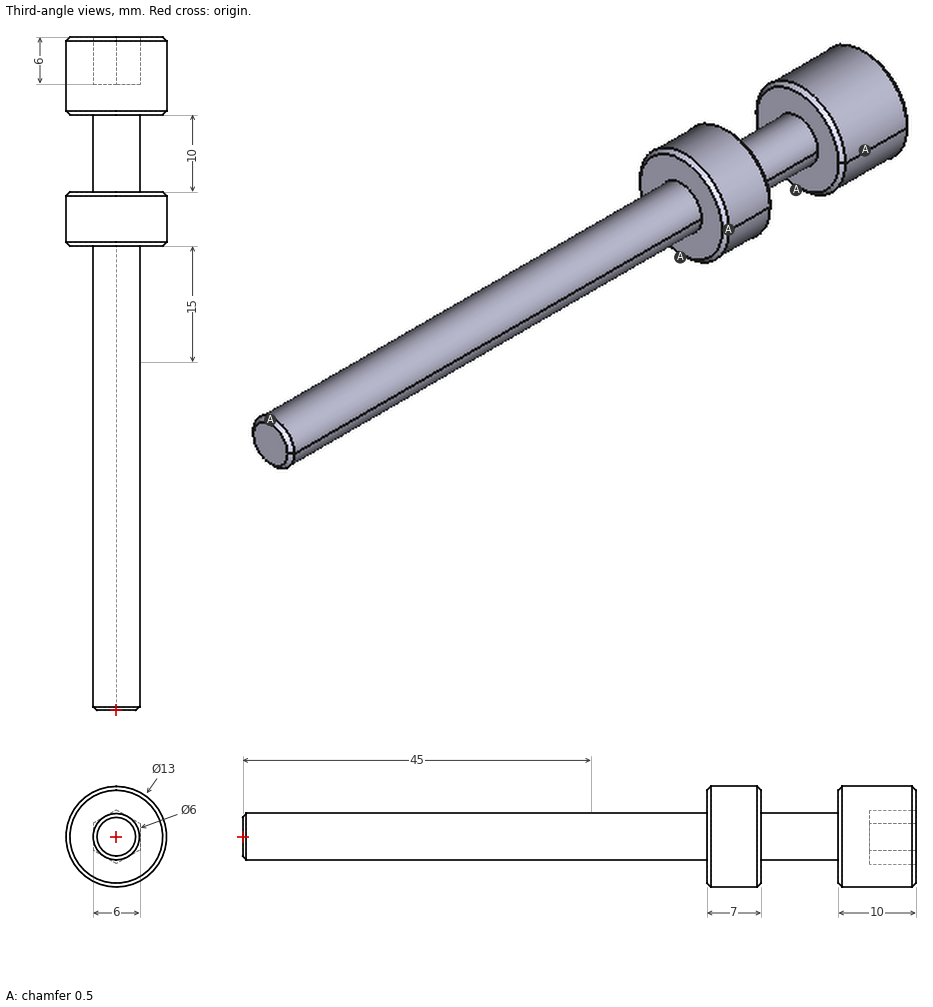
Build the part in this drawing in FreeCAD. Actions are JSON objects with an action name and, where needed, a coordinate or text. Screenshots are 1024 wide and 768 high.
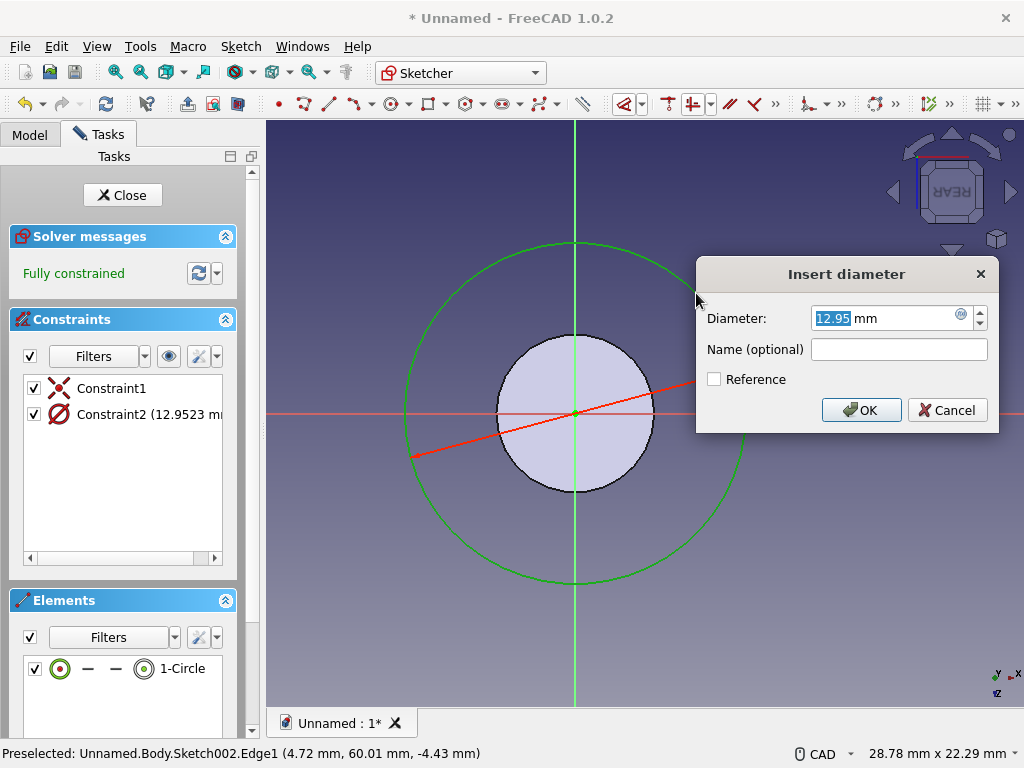
{"action": "type", "text": "13"}
{"action": "key", "text": "Return"}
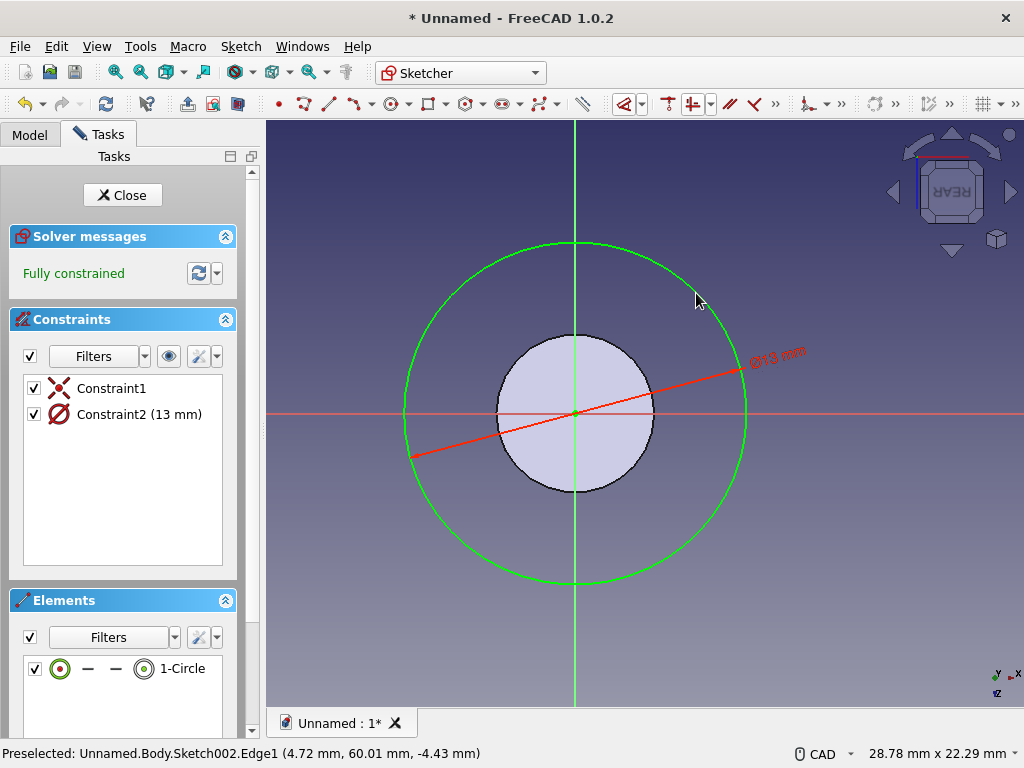
{"action": "left_click", "coordinate": [123, 195]}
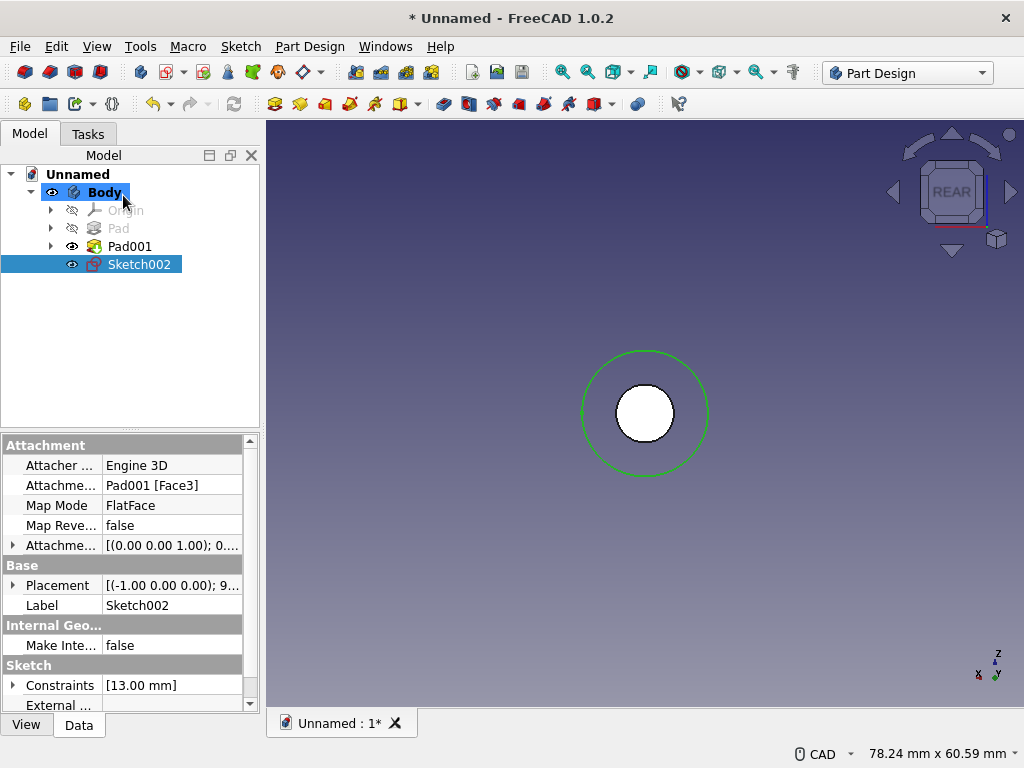
{"action": "left_click", "coordinate": [275, 104]}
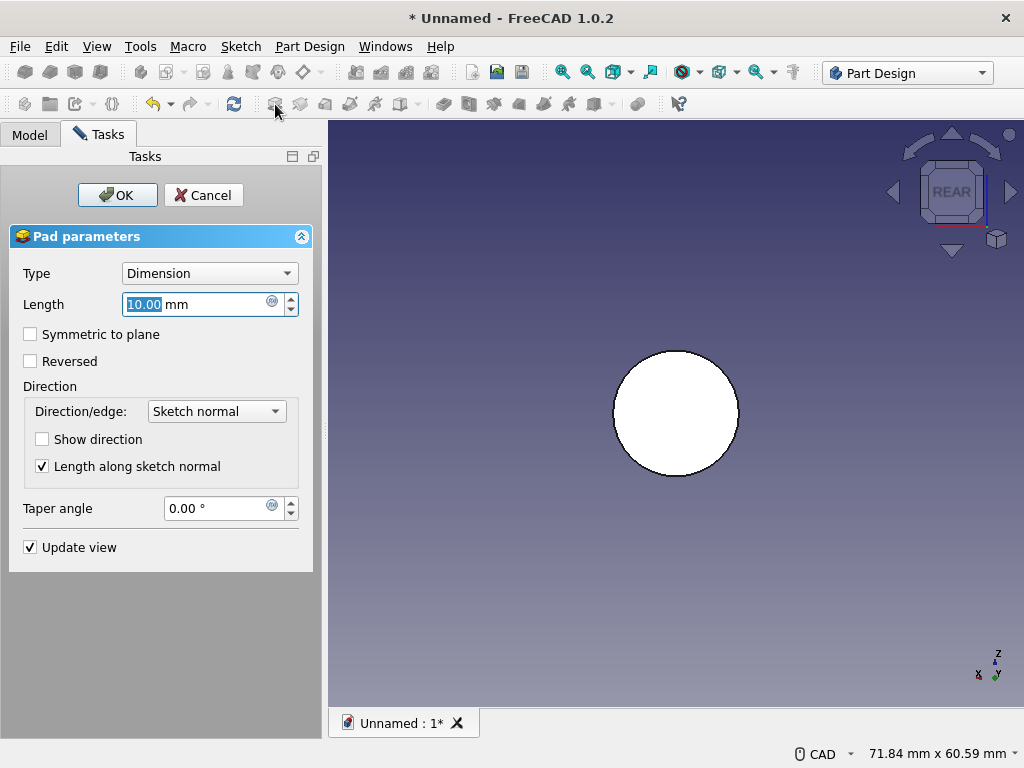
{"action": "type", "text": "7"}
{"action": "key", "text": "Tab"}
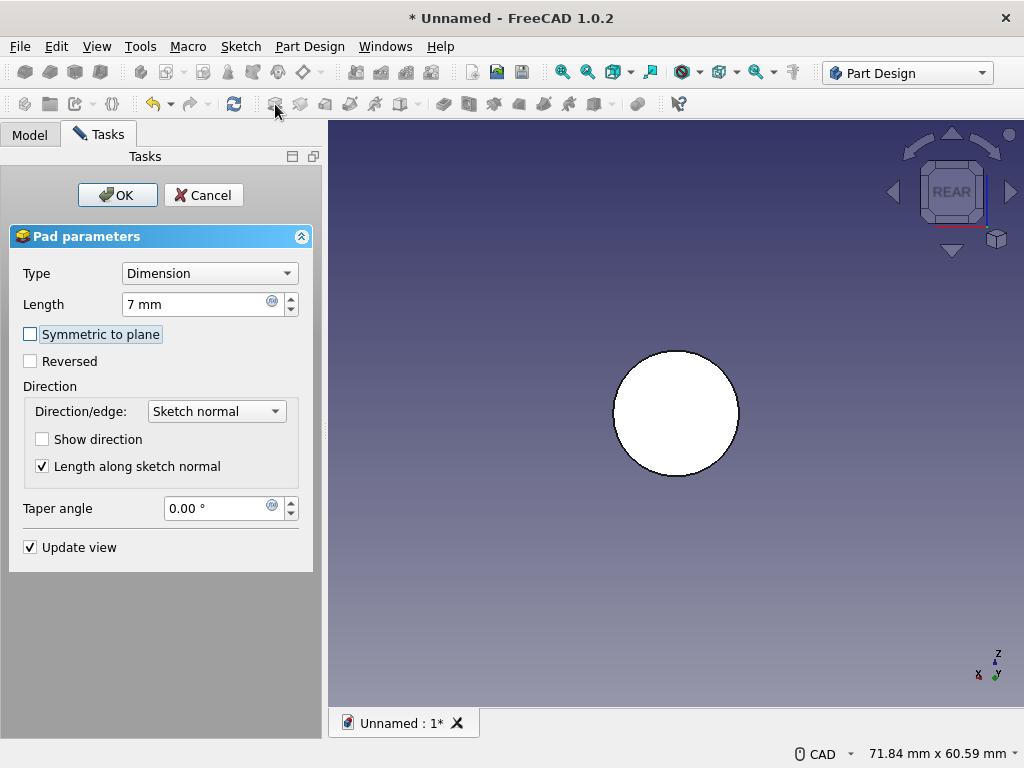
{"action": "left_click", "coordinate": [118, 195]}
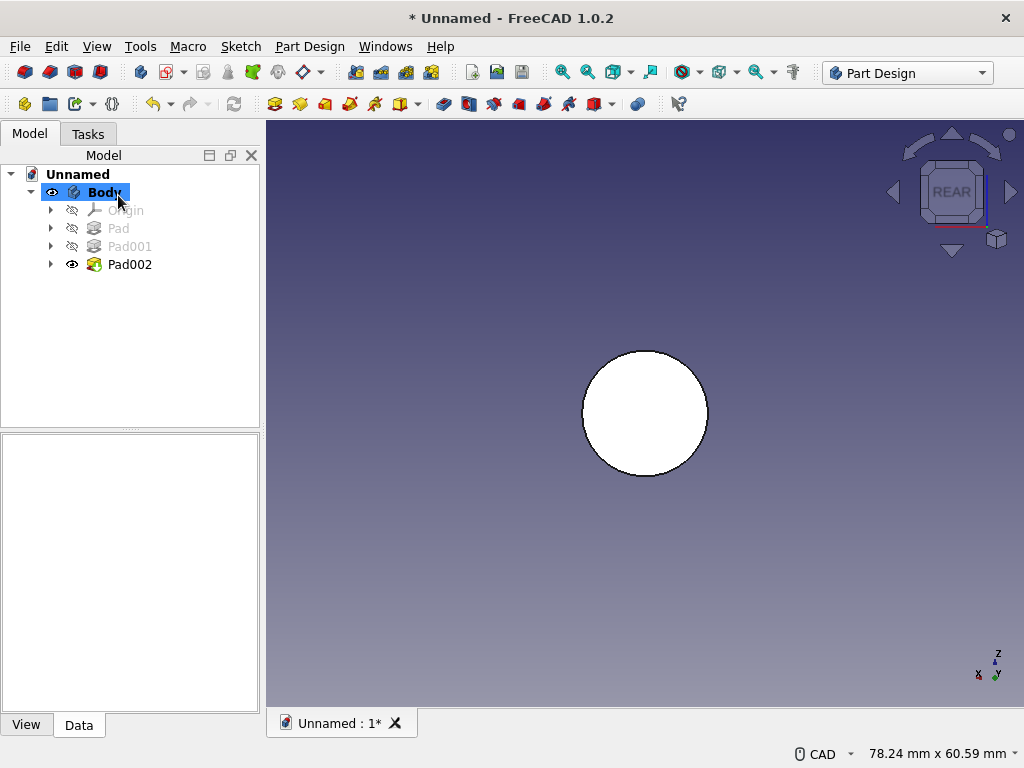
{"action": "key", "text": "v f"}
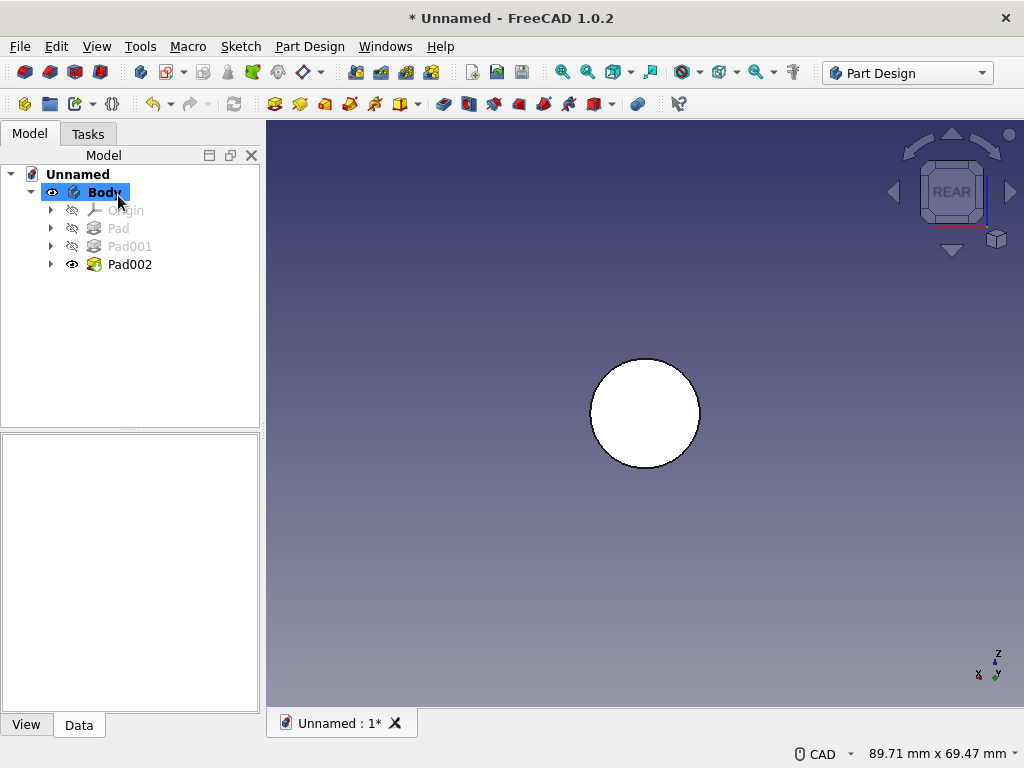
{"action": "left_click", "coordinate": [645, 412]}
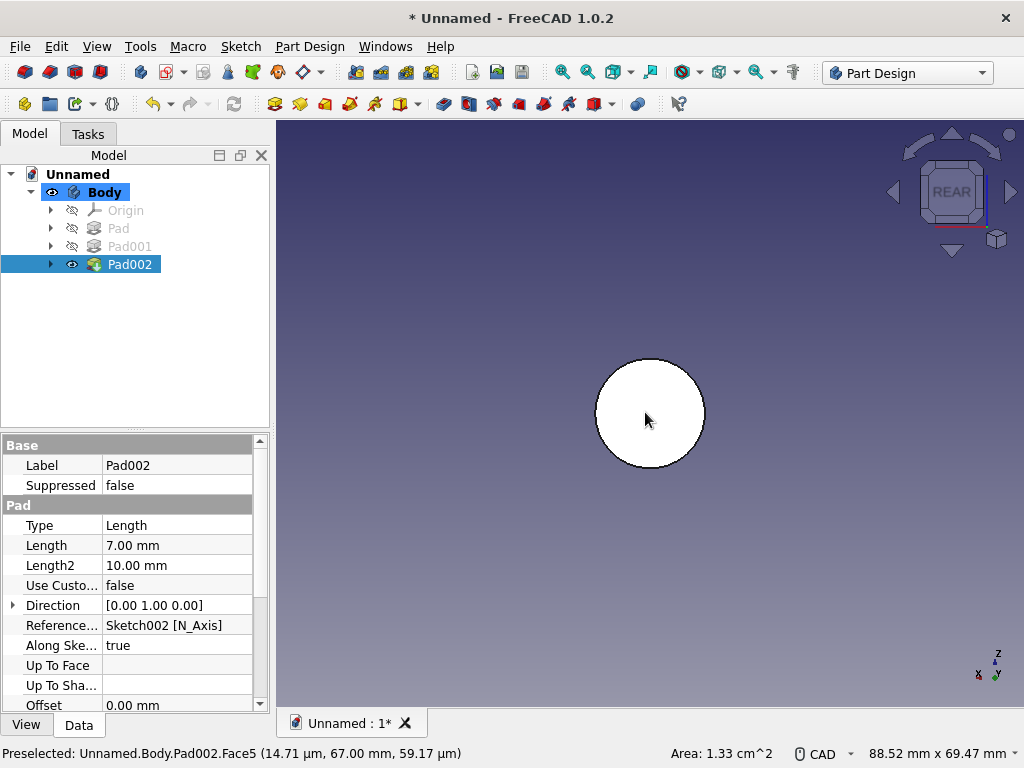
{"action": "left_click", "coordinate": [166, 72]}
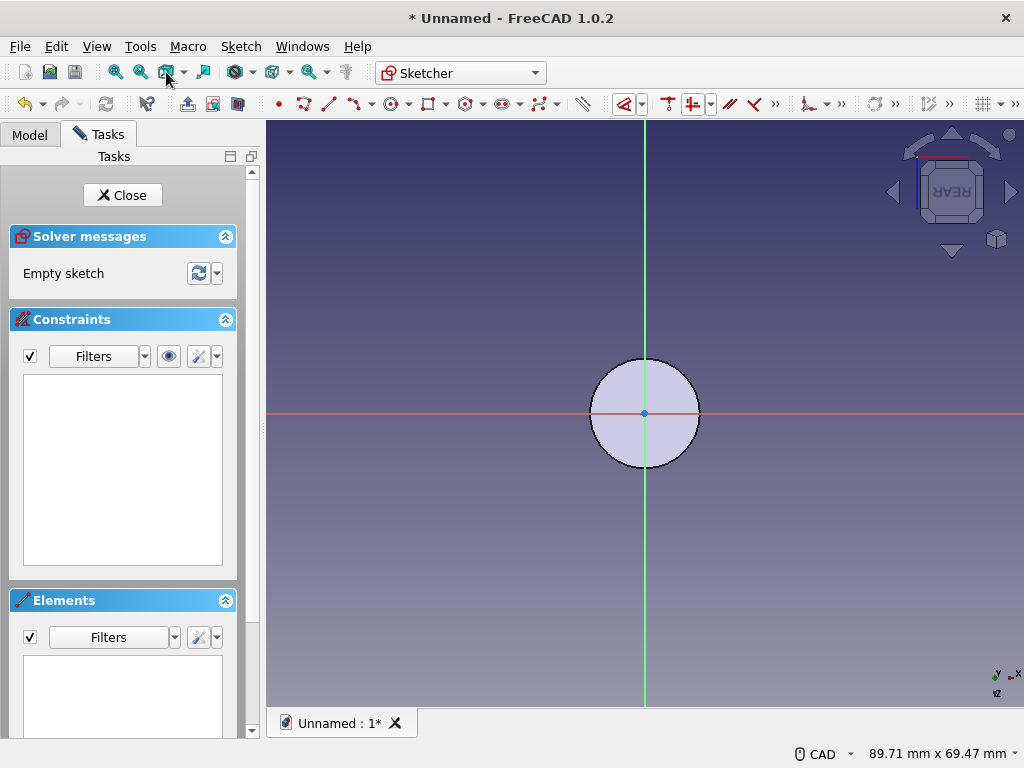
{"action": "scroll", "coordinate": [656, 413], "scroll_direction": "up", "scroll_amount": 10}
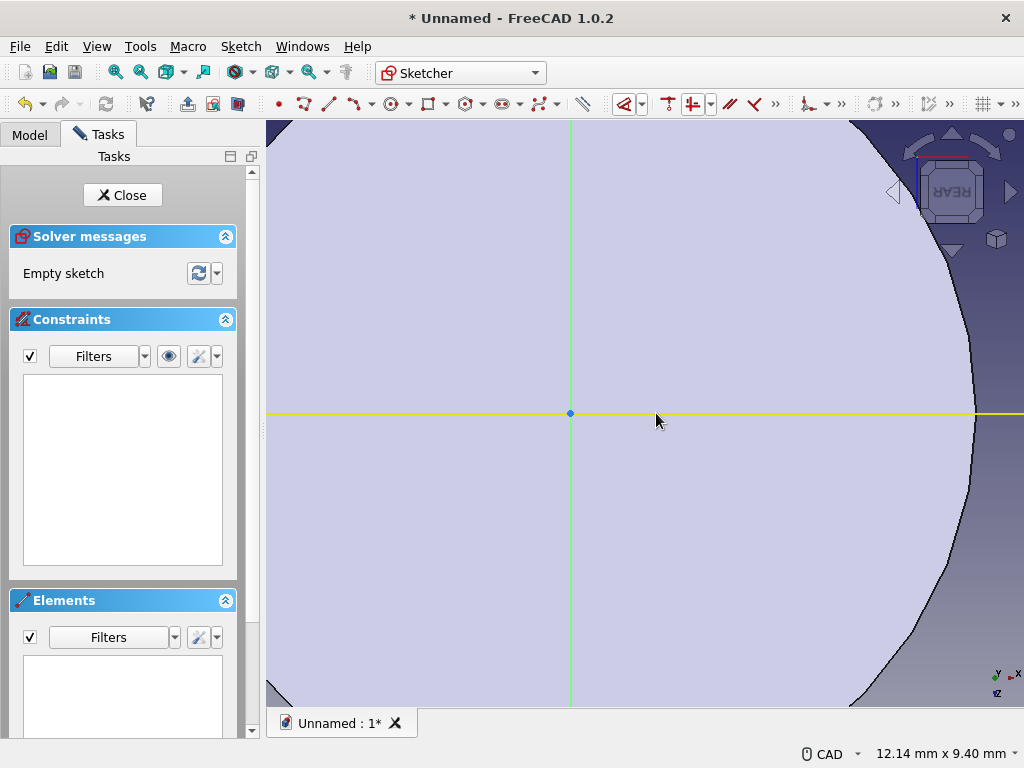
{"action": "left_click", "coordinate": [390, 104]}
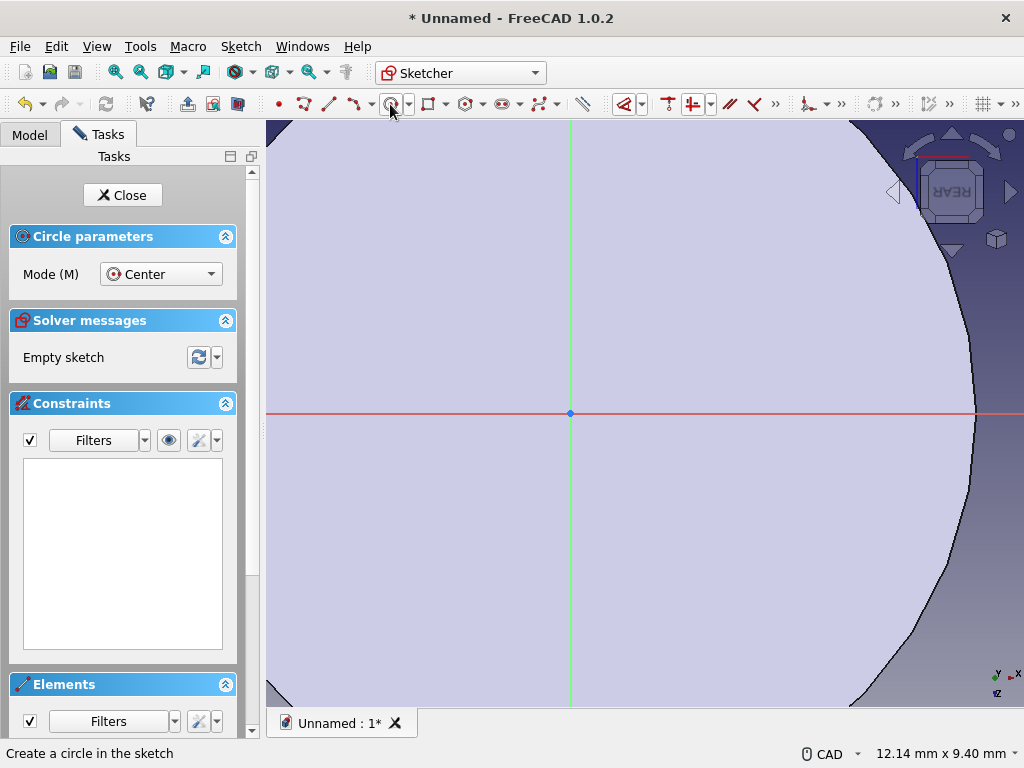
{"action": "left_click", "coordinate": [571, 413]}
{"action": "left_click", "coordinate": [703, 281]}
{"action": "key", "text": "Escape"}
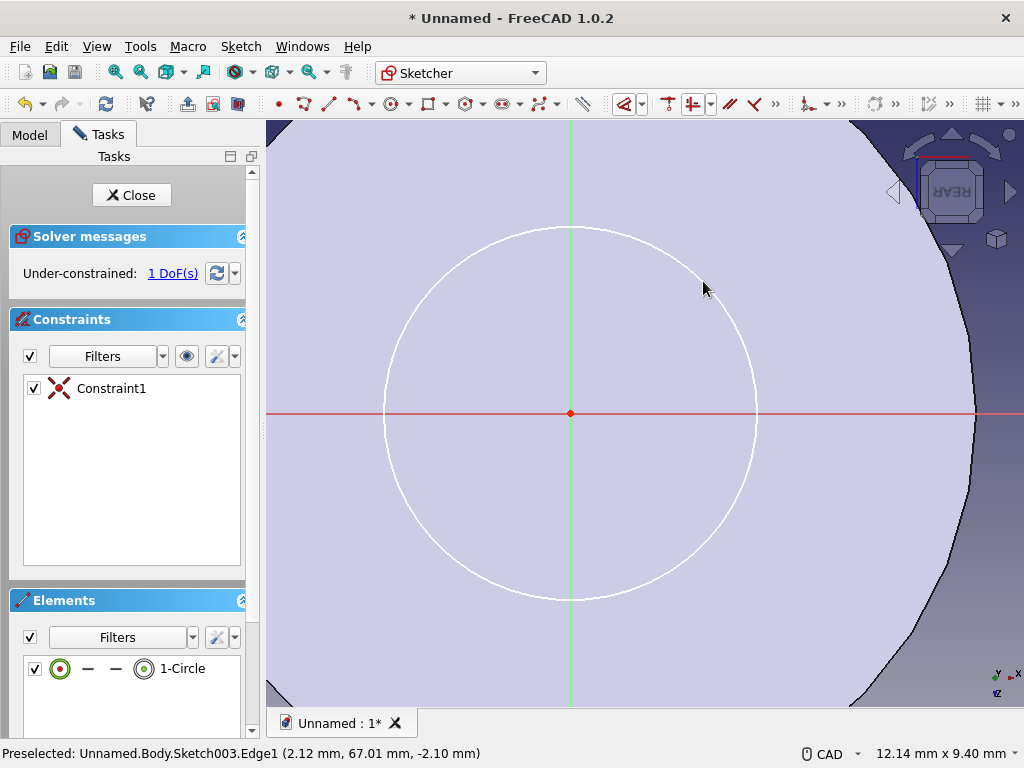
{"action": "left_click", "coordinate": [702, 281]}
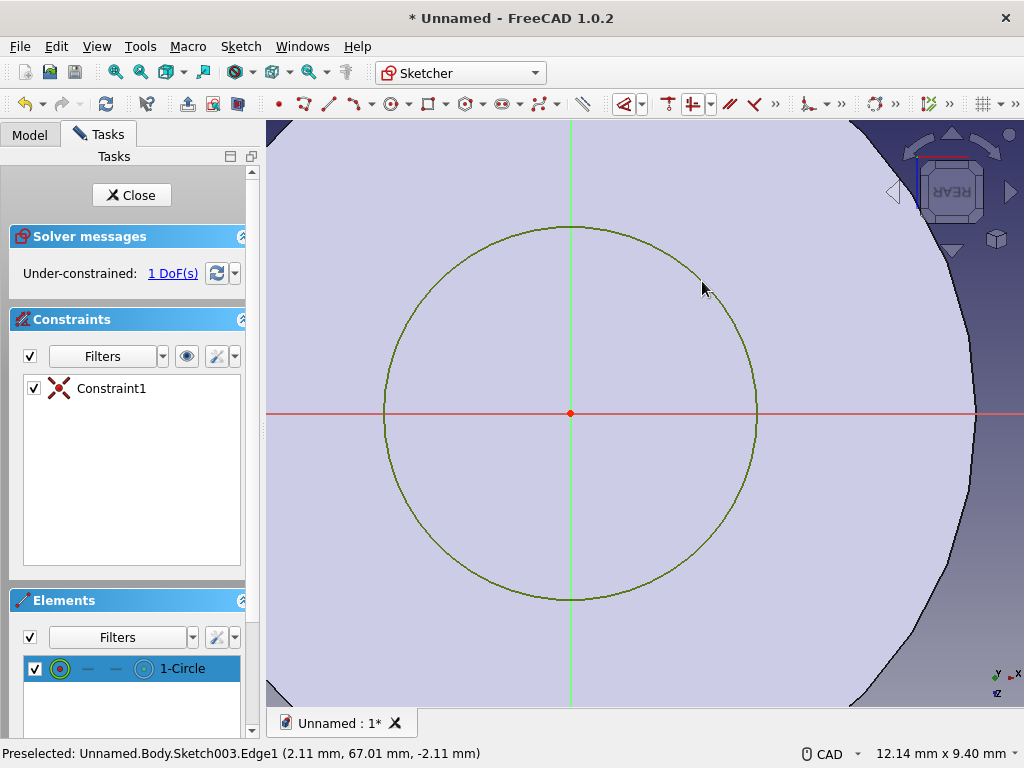
{"action": "key", "text": "k o"}